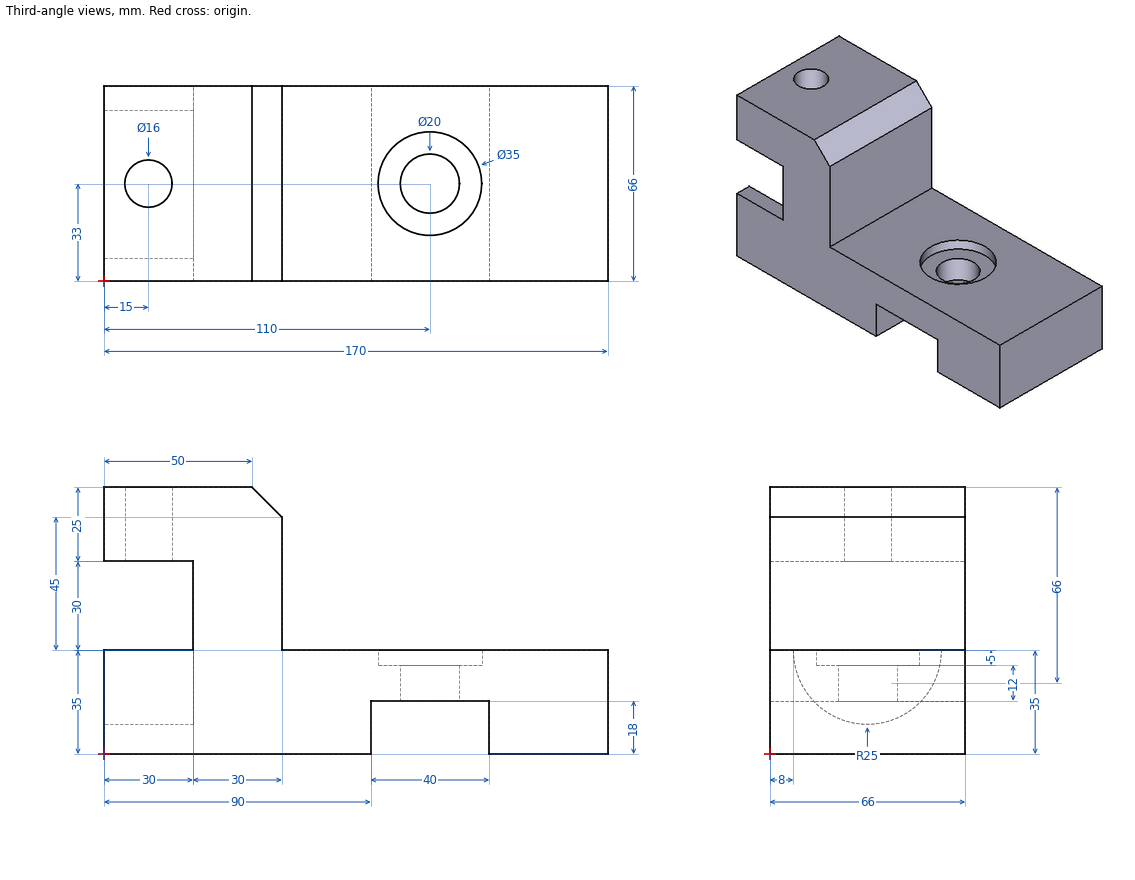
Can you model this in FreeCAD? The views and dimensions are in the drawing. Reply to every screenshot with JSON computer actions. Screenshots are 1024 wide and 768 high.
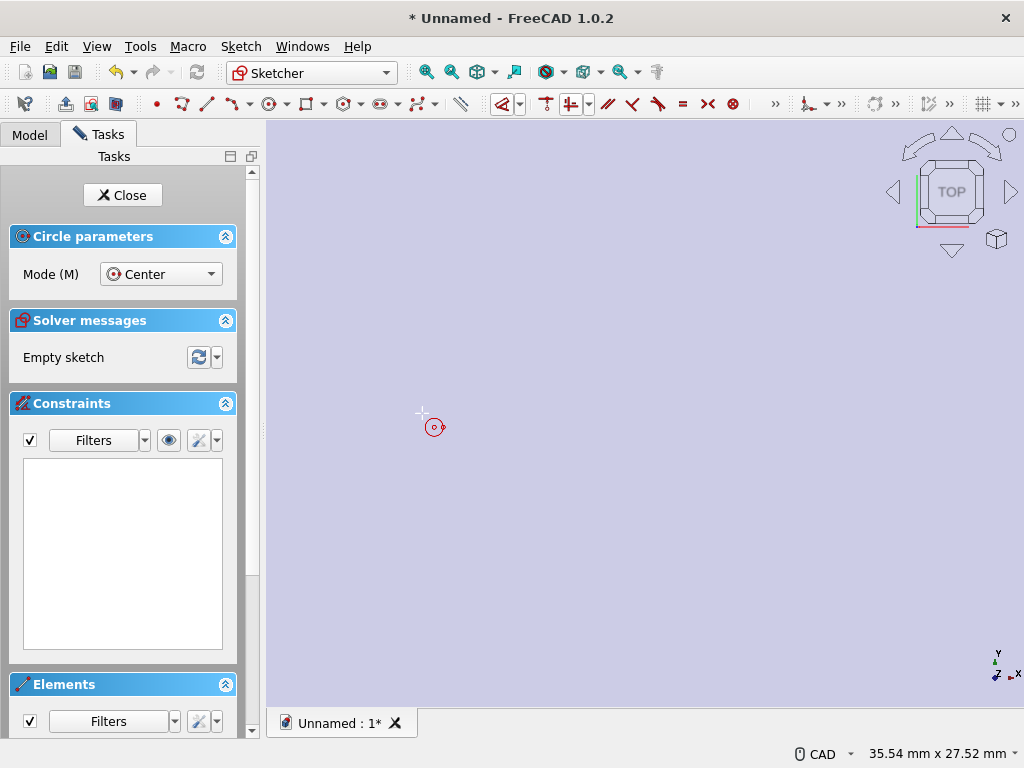
{"action": "left_click", "coordinate": [575, 413]}
{"action": "mouse_move", "coordinate": [696, 293]}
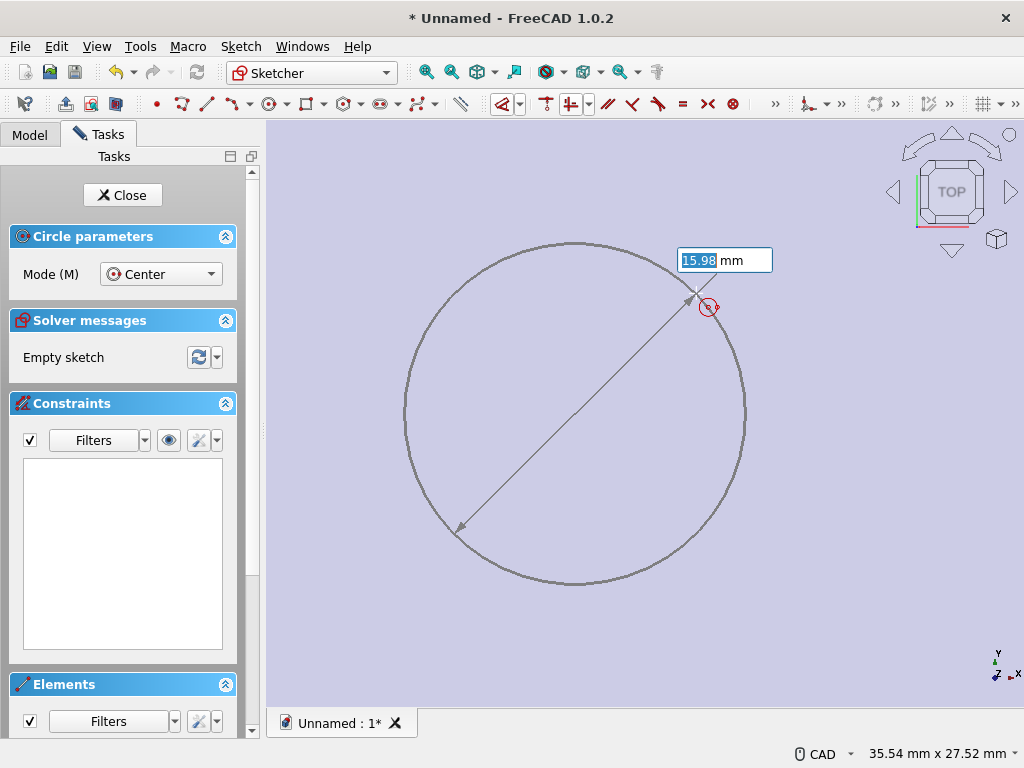
{"action": "type", "text": "16"}
{"action": "key", "text": "Return"}
{"action": "key", "text": "Escape"}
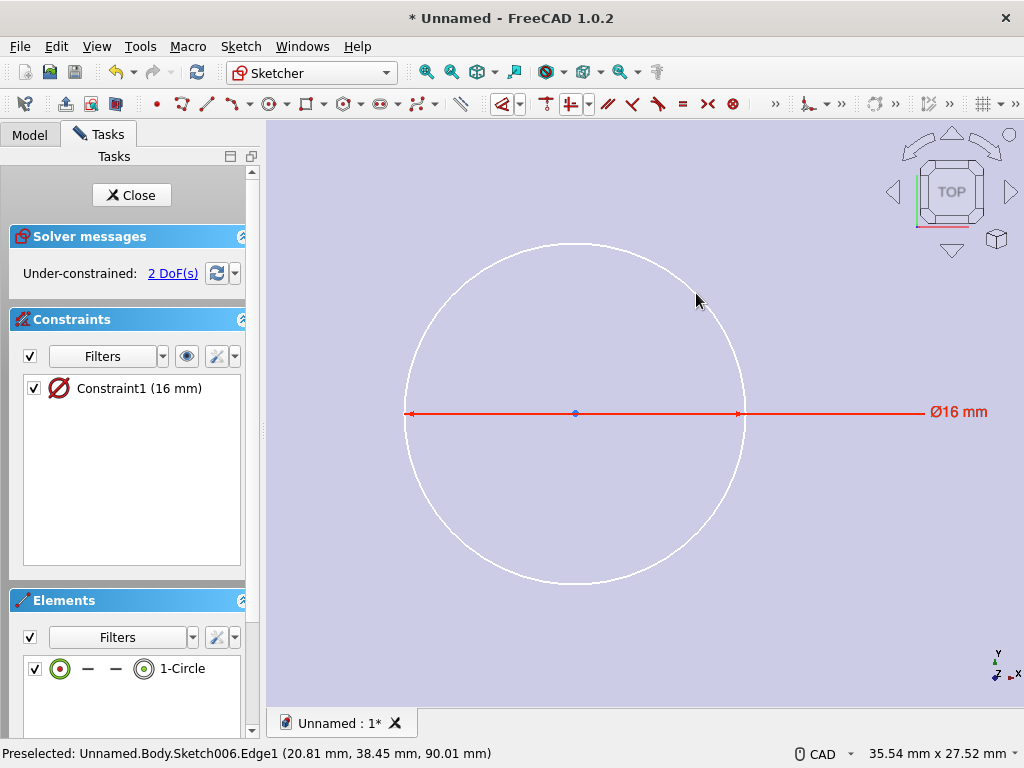
{"action": "left_click", "coordinate": [575, 414]}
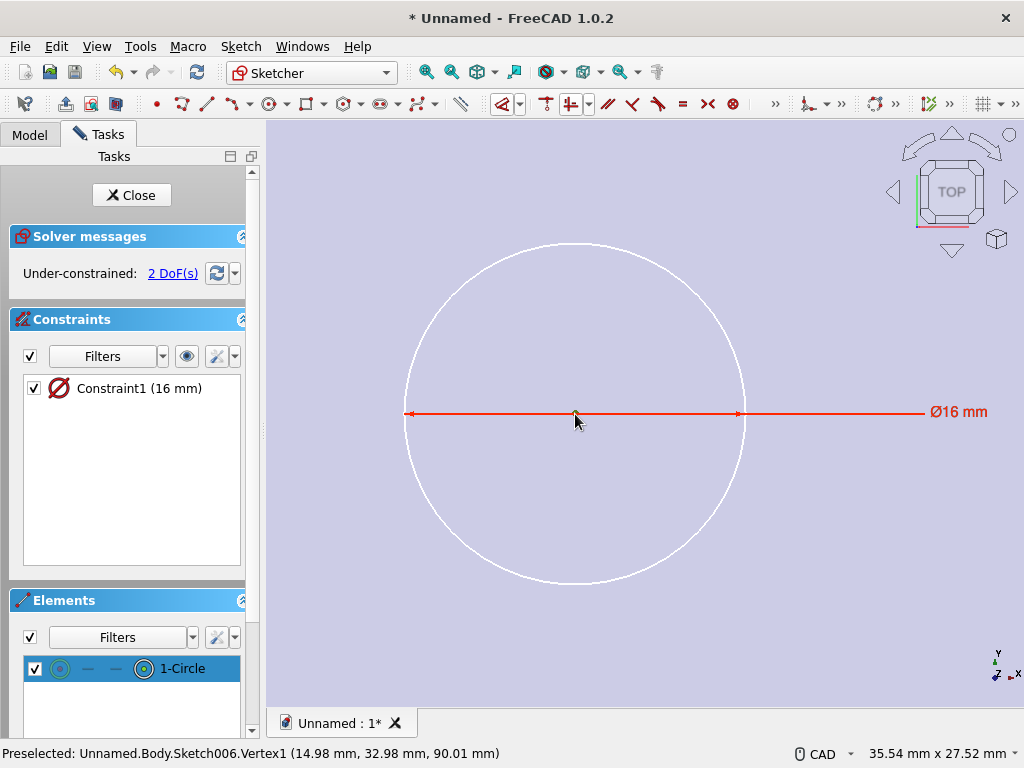
{"action": "key", "text": "l"}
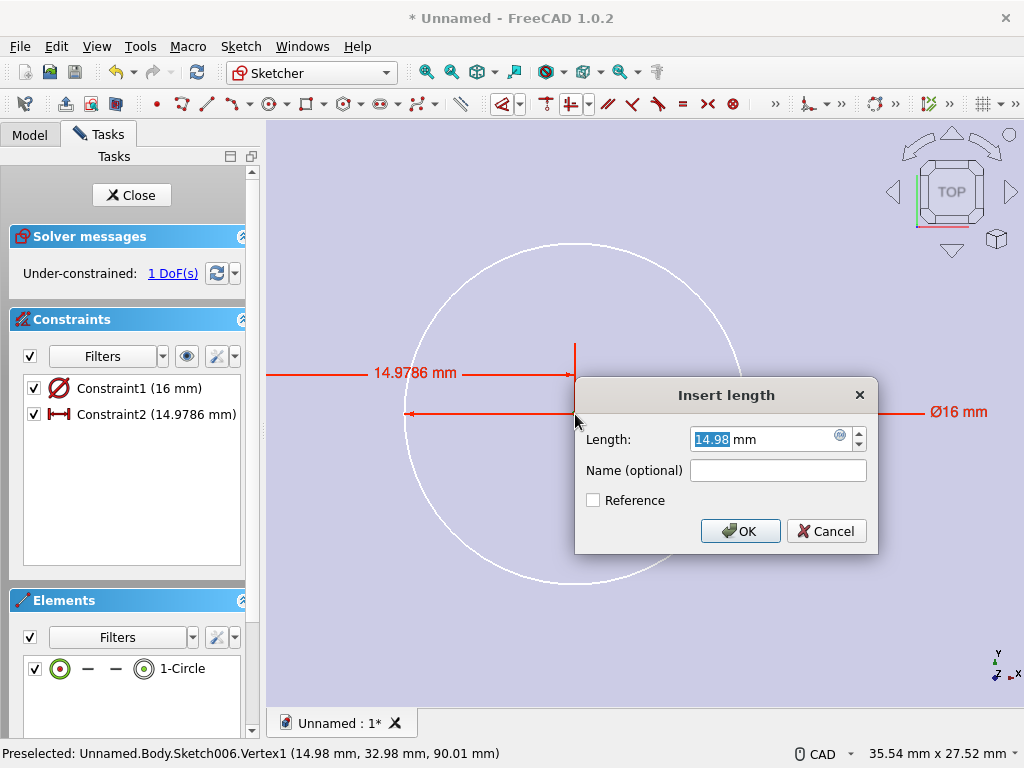
{"action": "type", "text": "15"}
{"action": "key", "text": "Return"}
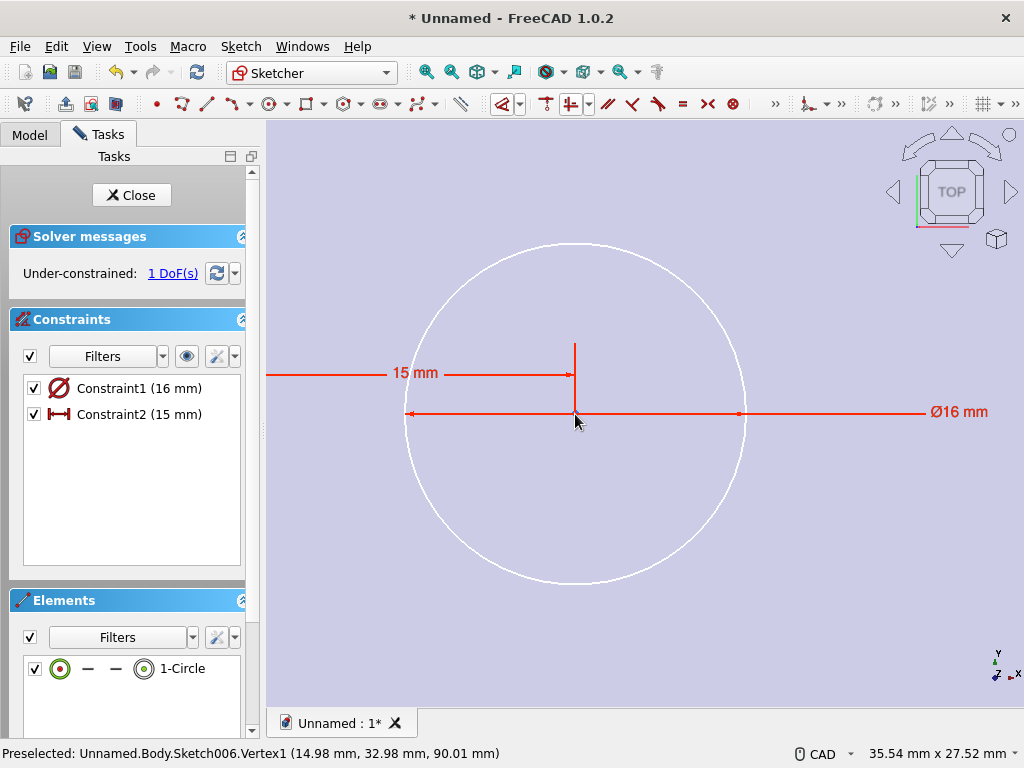
{"action": "left_click", "coordinate": [575, 414]}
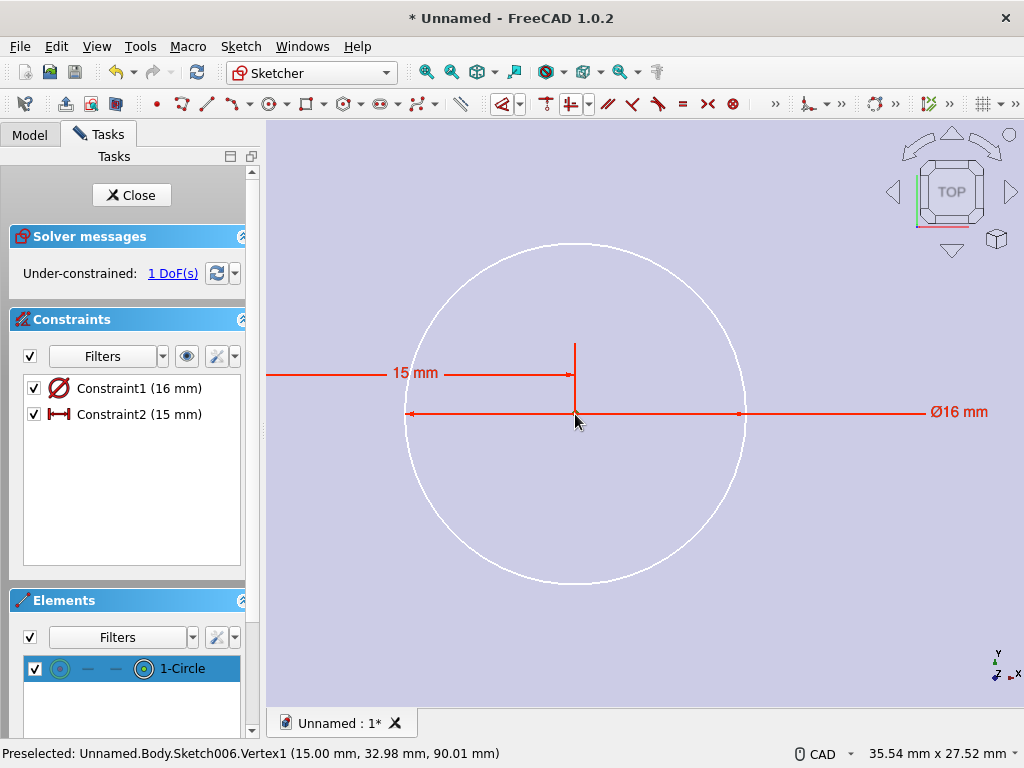
{"action": "key", "text": "i"}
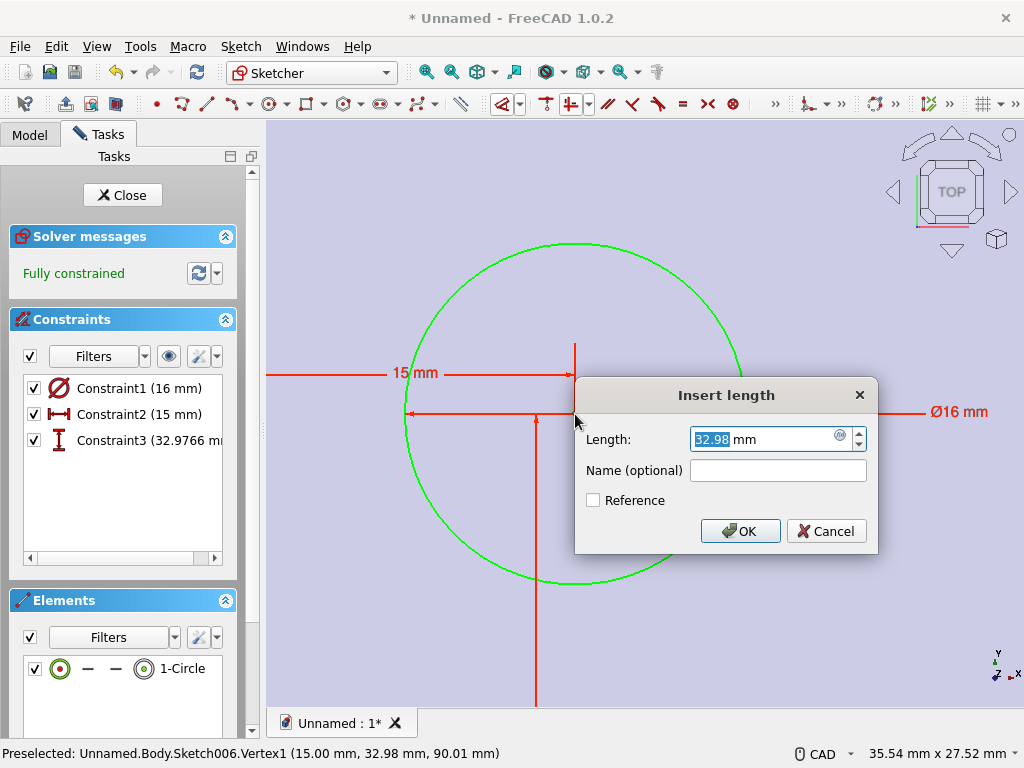
{"action": "type", "text": "33"}
{"action": "key", "text": "Return"}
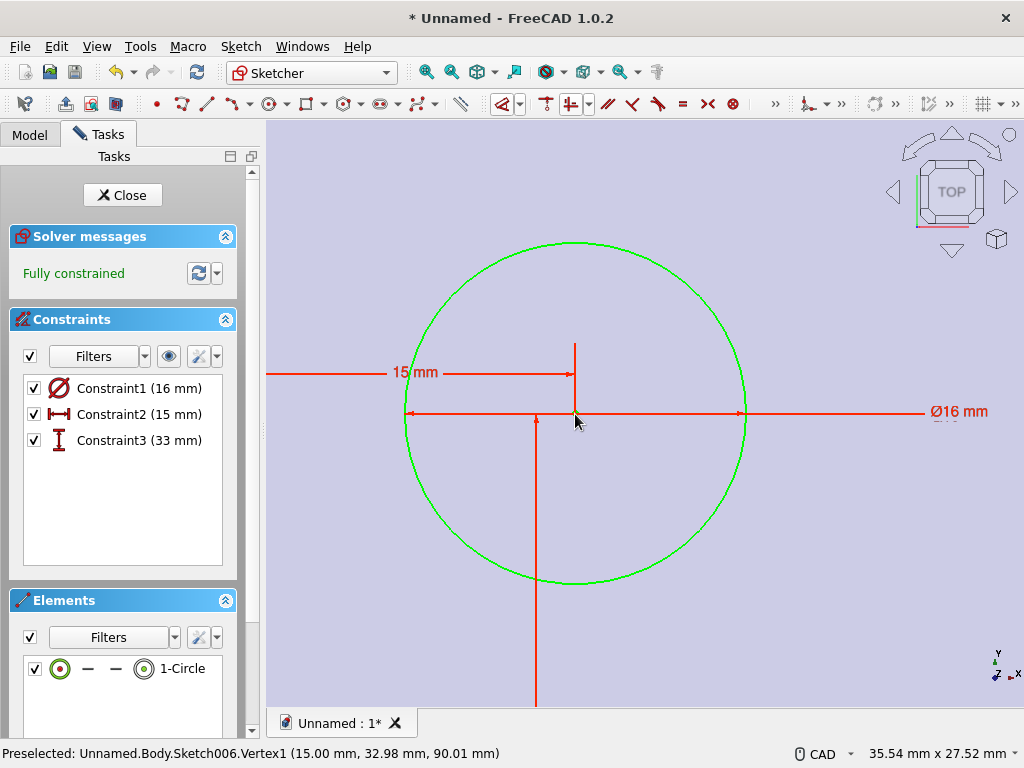
{"action": "left_click", "coordinate": [123, 195]}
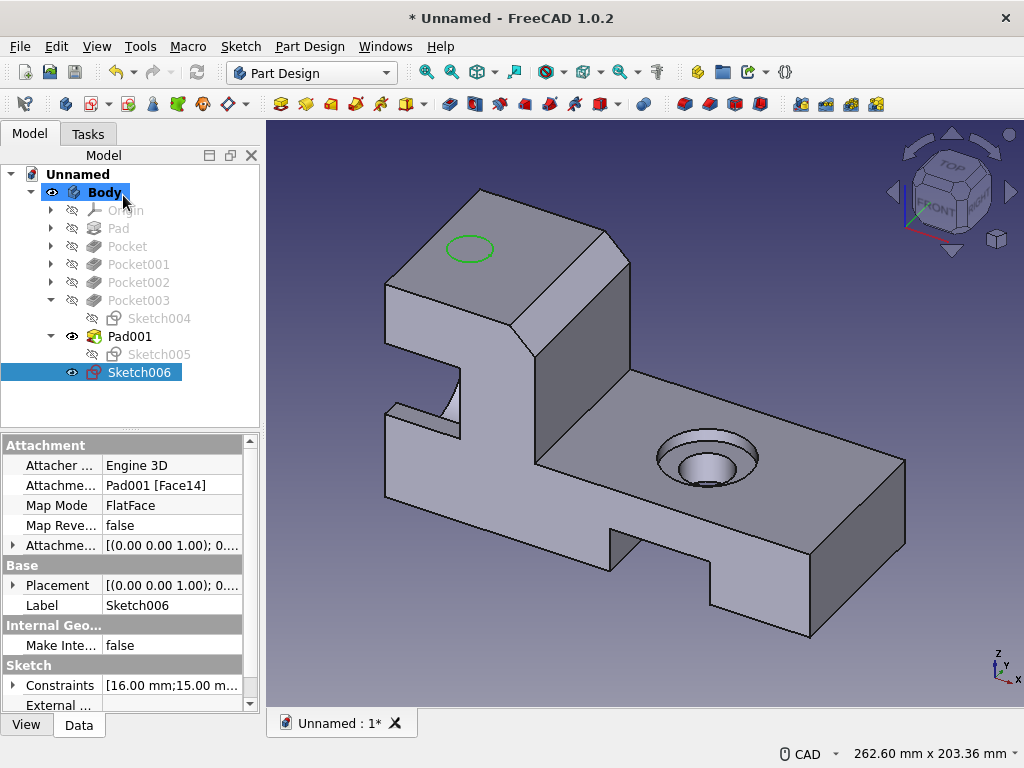
{"action": "left_click", "coordinate": [450, 104]}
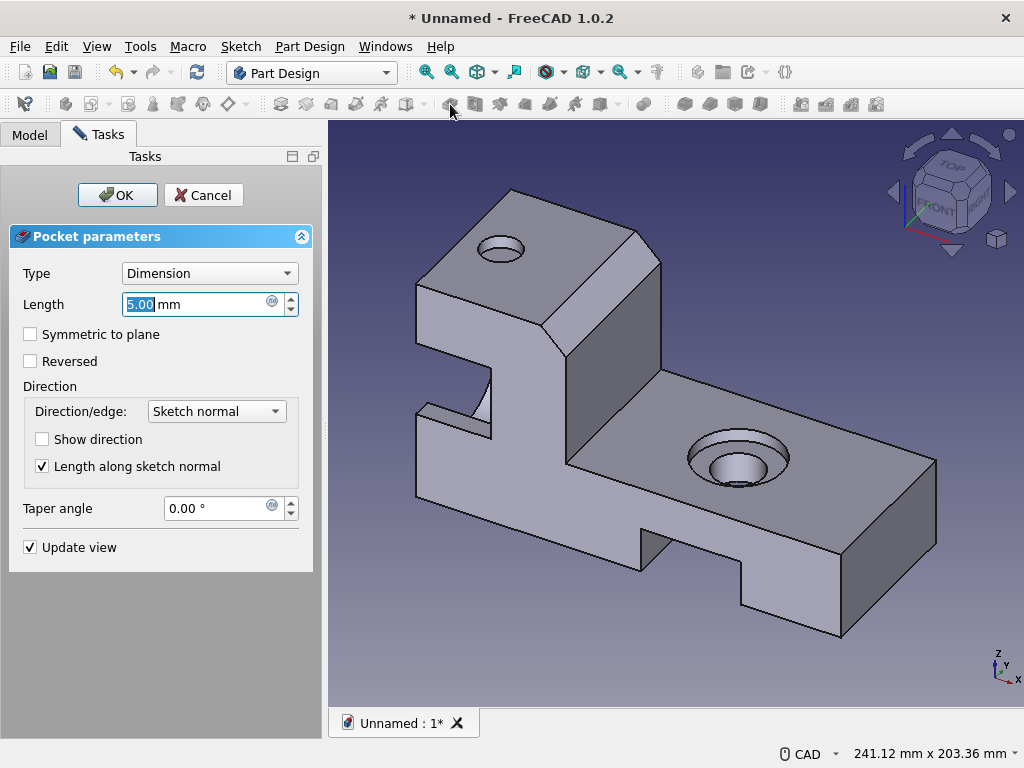
{"action": "type", "text": "66"}
{"action": "key", "text": "Tab"}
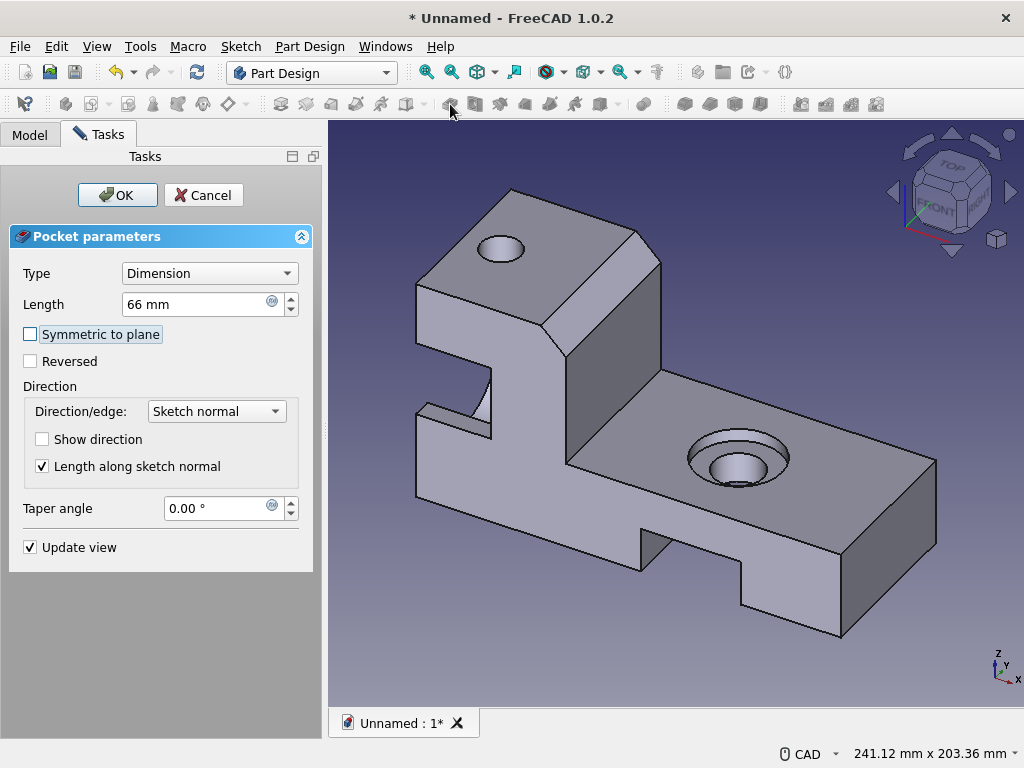
{"action": "left_click", "coordinate": [118, 195]}